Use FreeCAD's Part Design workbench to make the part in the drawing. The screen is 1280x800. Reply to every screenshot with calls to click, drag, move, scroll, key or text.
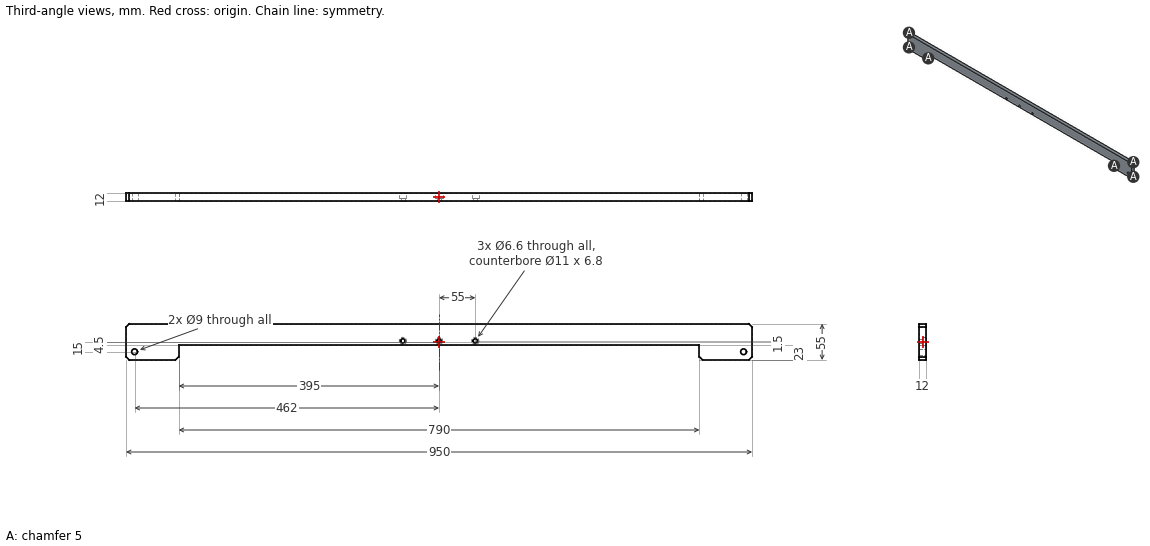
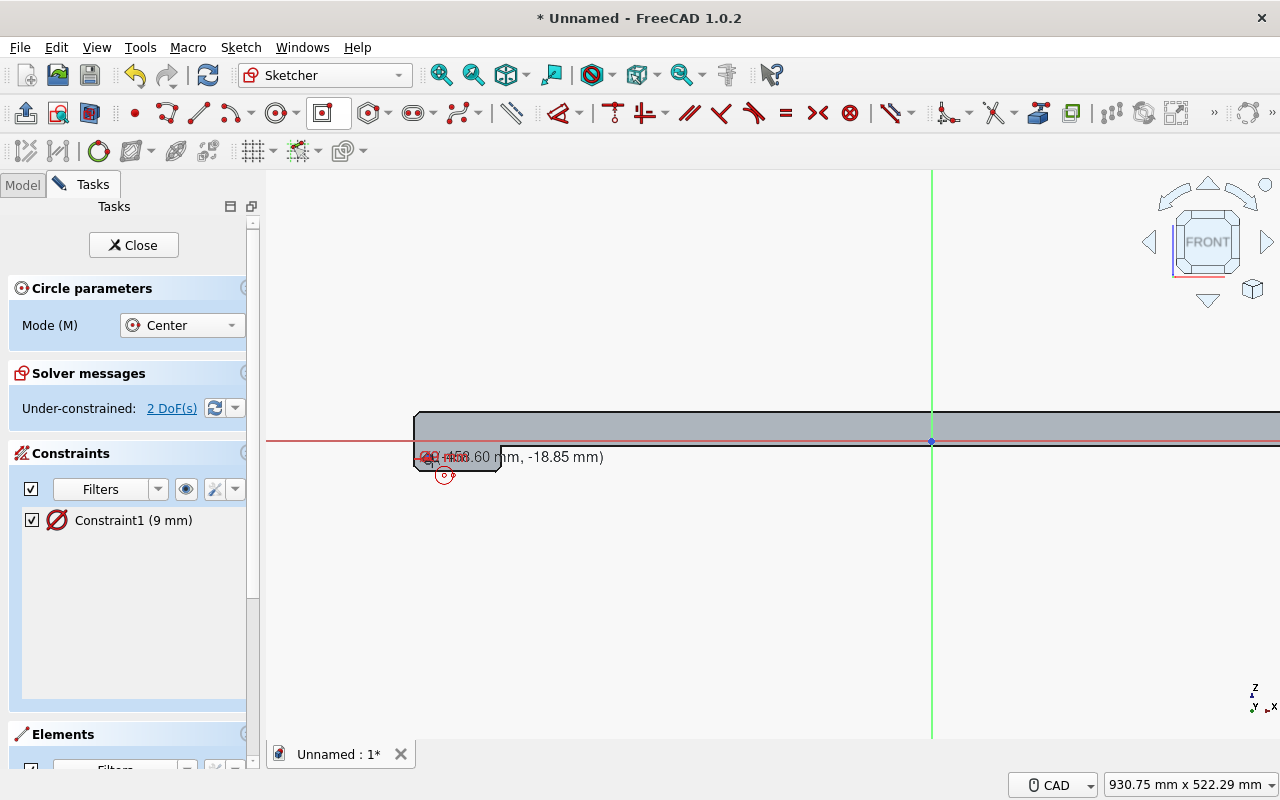
scroll(428, 457, down, 3)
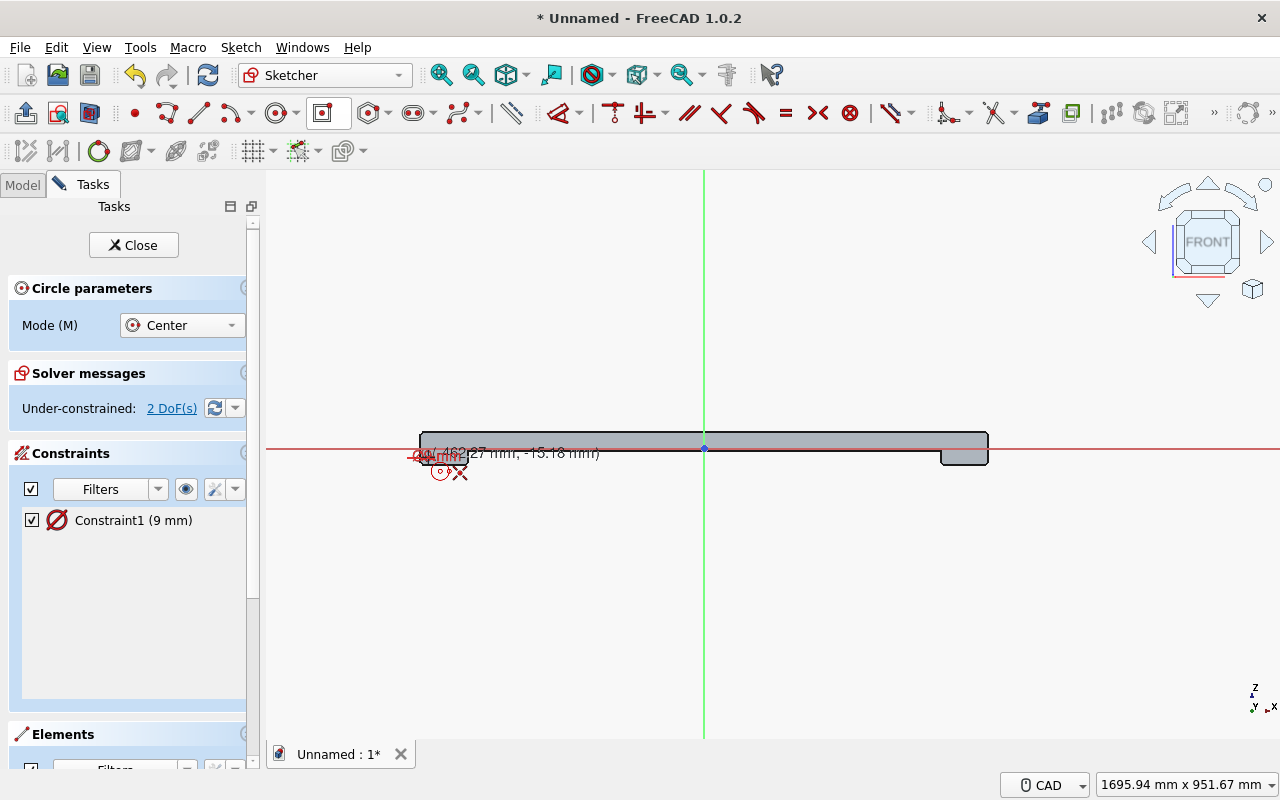
scroll(981, 458, up, 11)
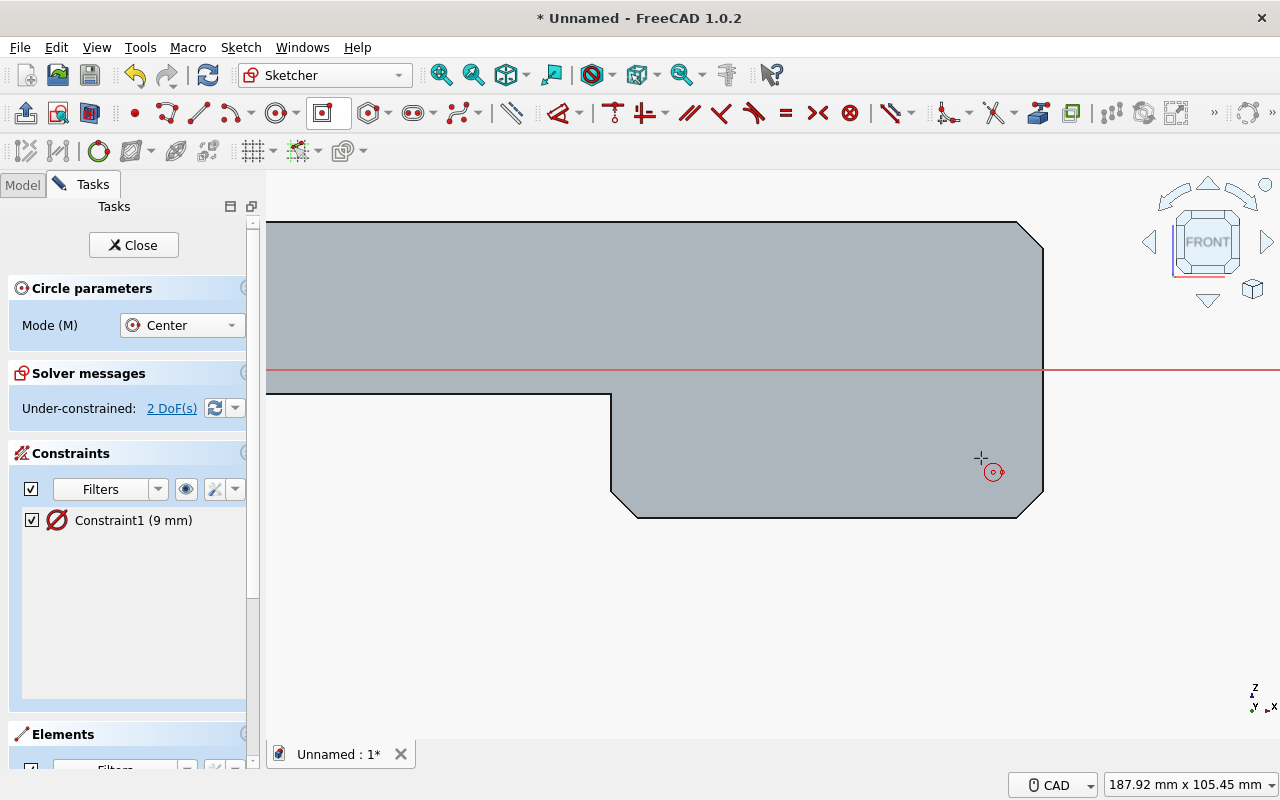
scroll(982, 458, down, 11)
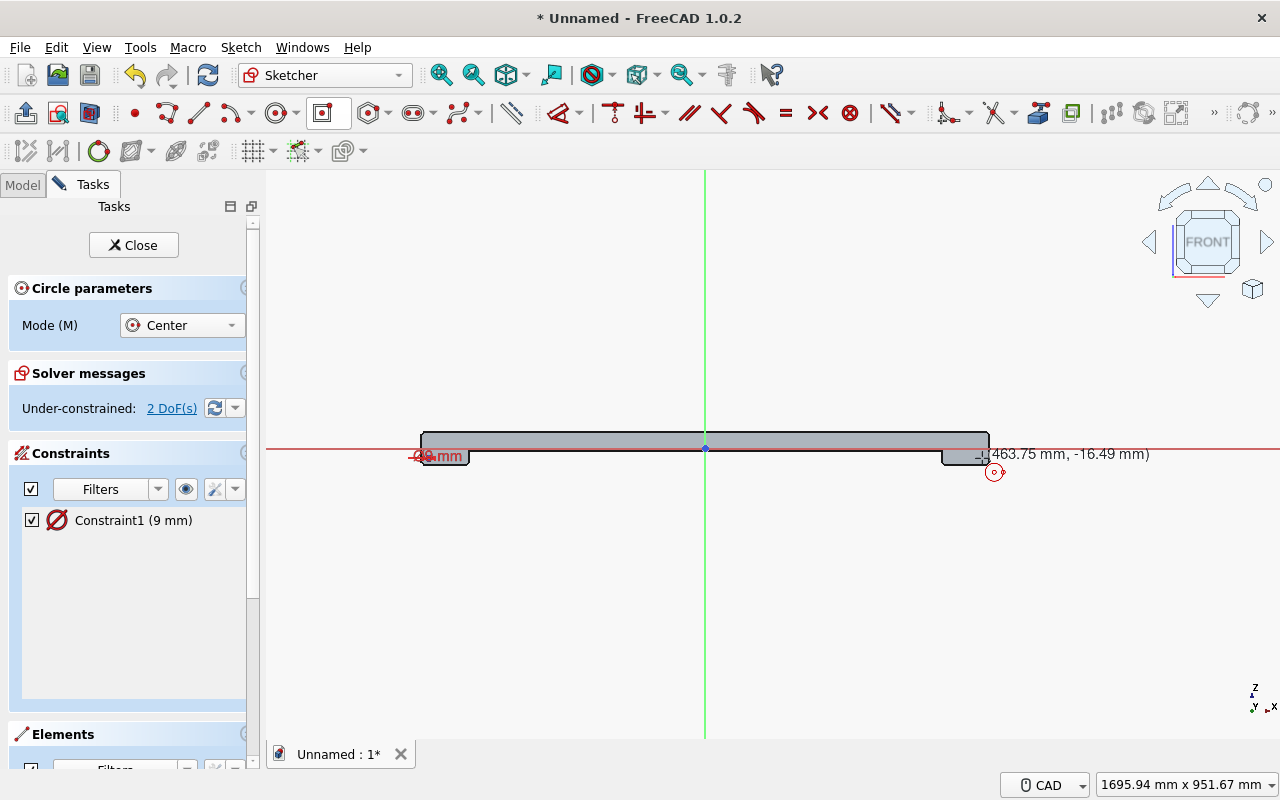
scroll(982, 458, up, 3)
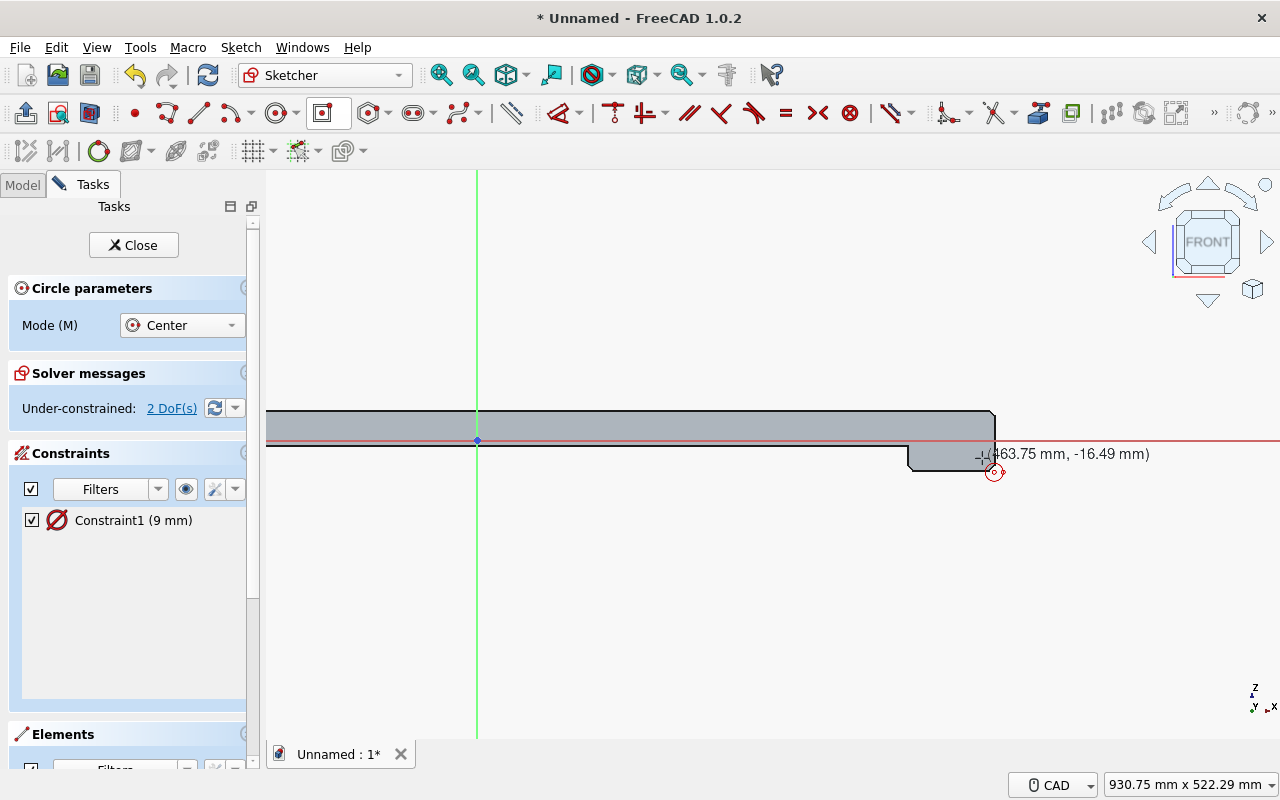
click(981, 457)
move(984, 460)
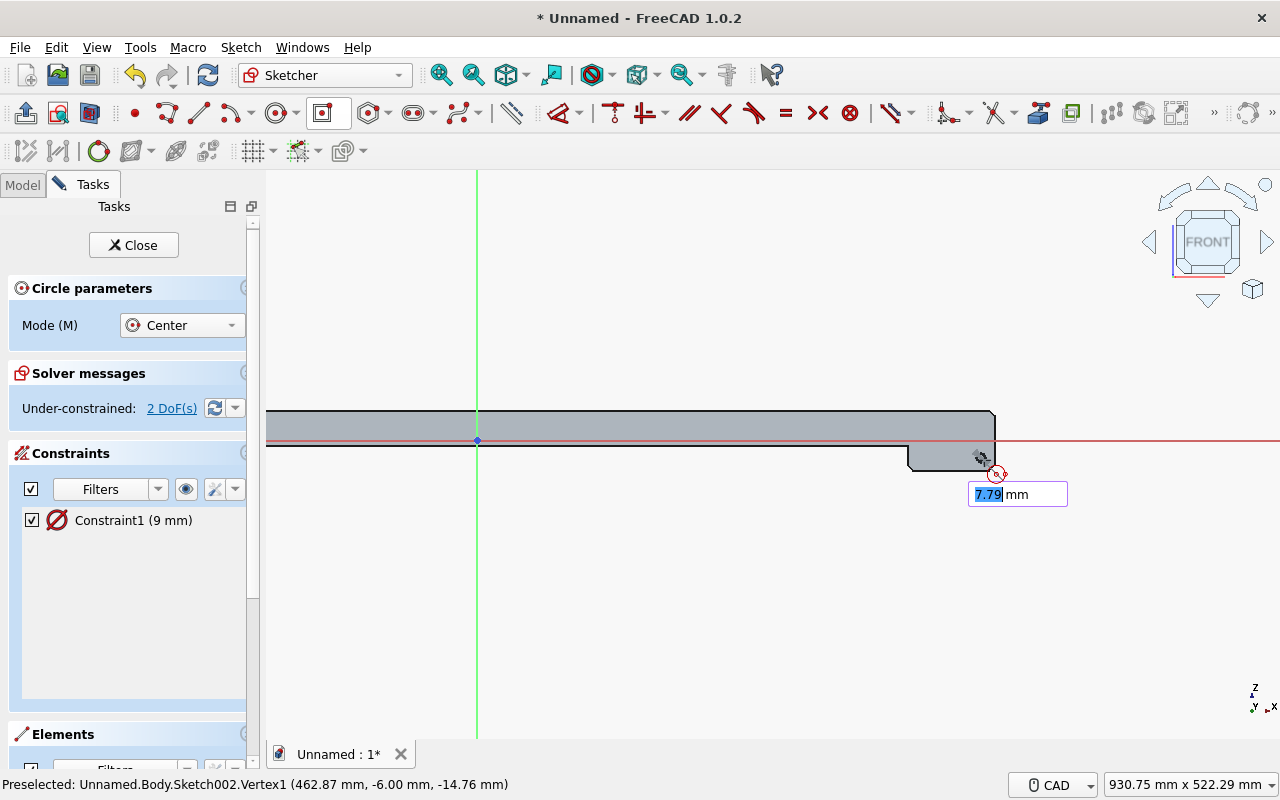
text(9)
key(Return)
key(Escape)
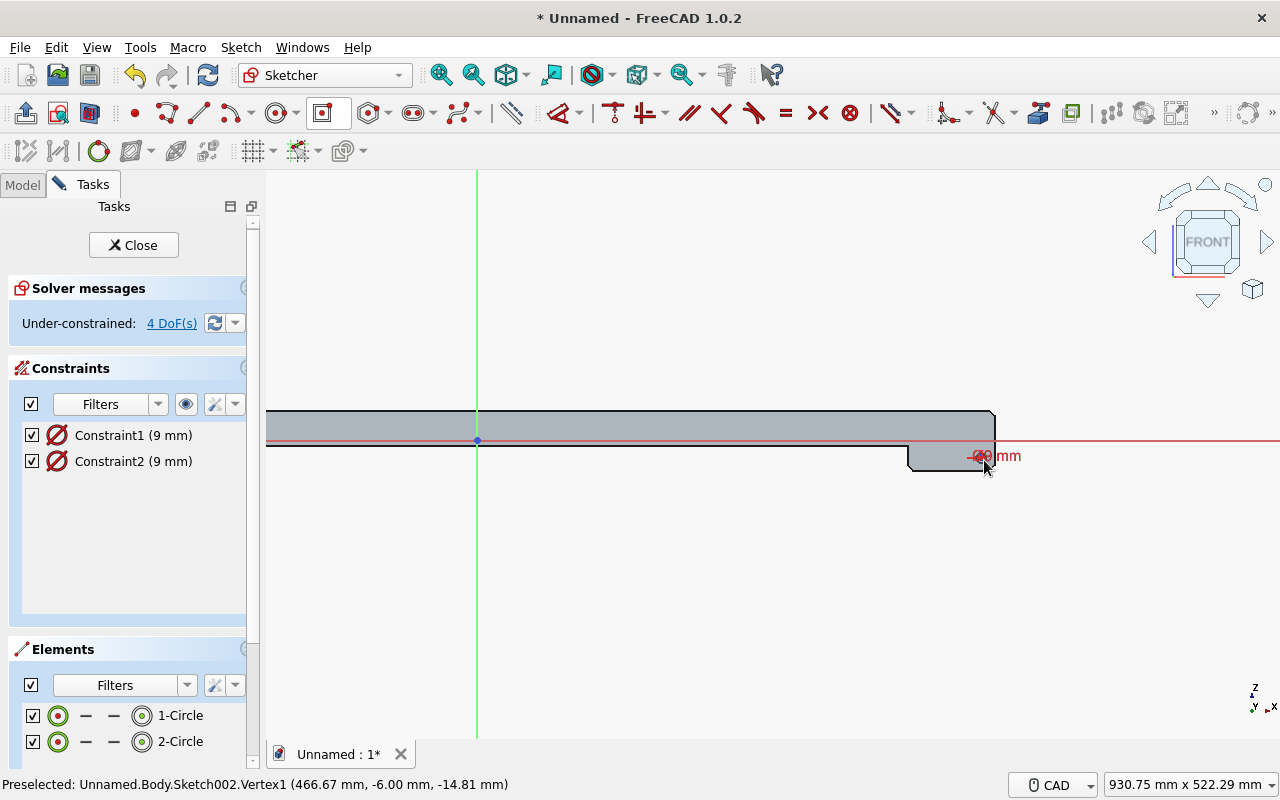
scroll(981, 458, down, 3)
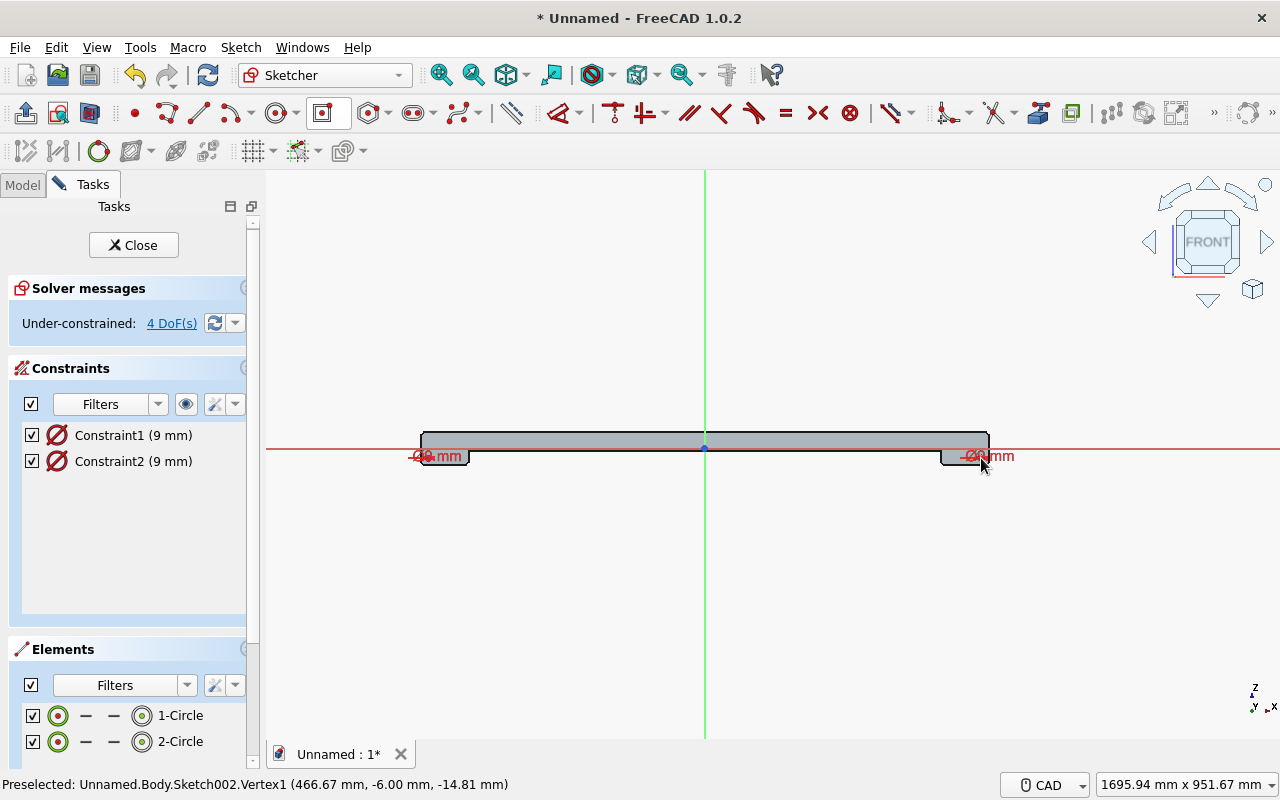
click(429, 458)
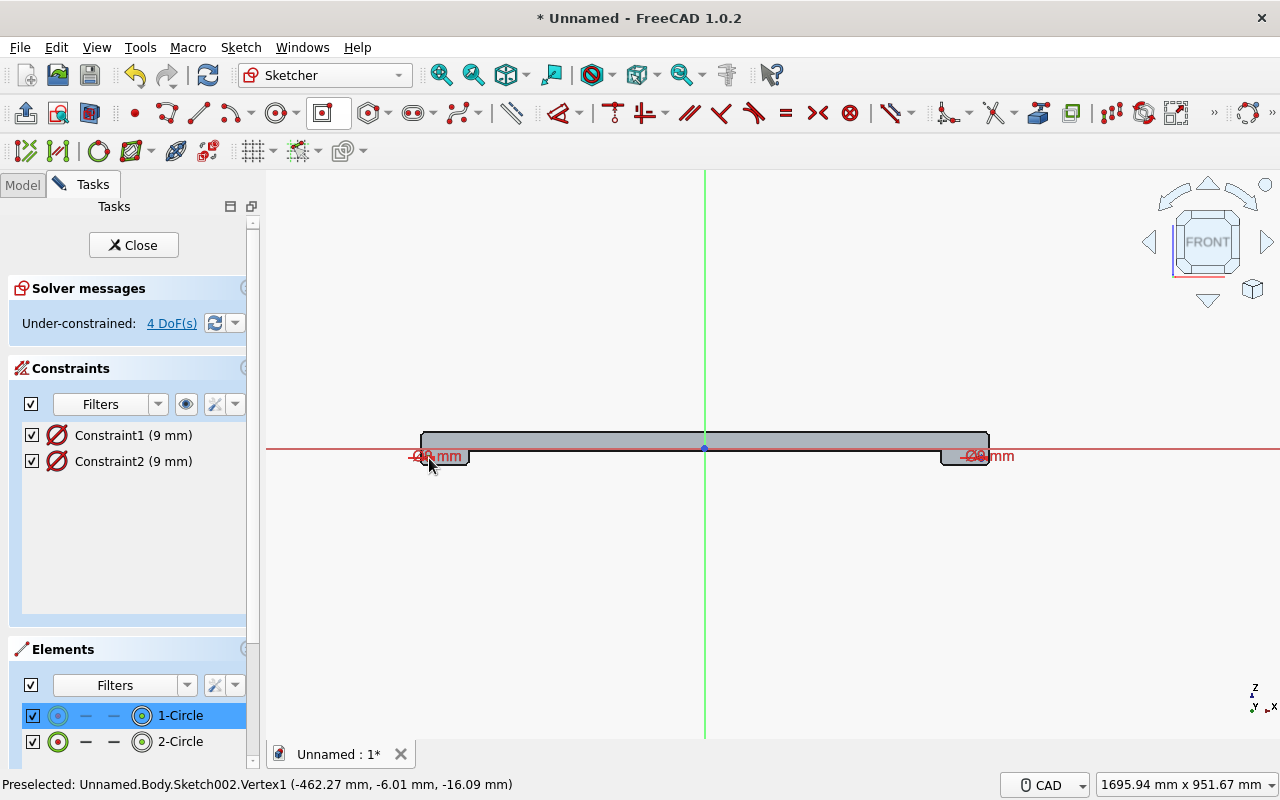
click(981, 458)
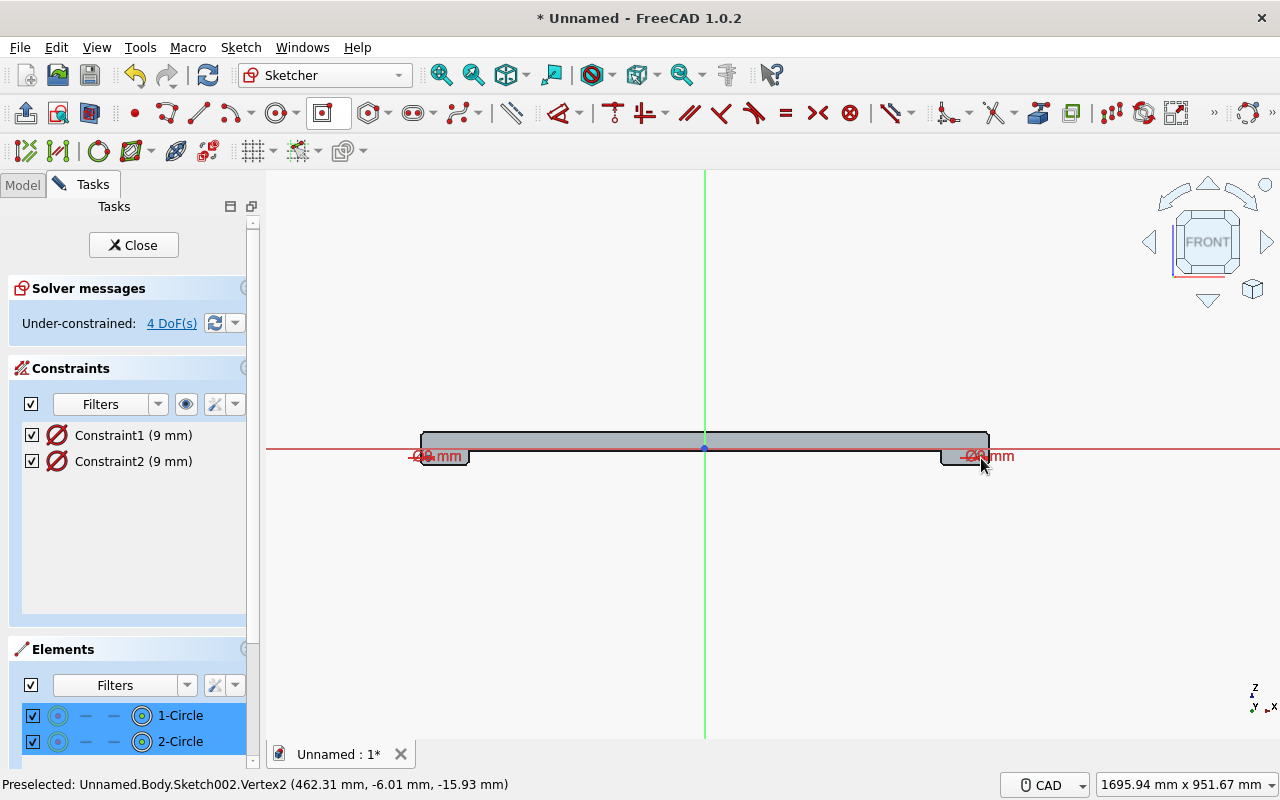
click(705, 674)